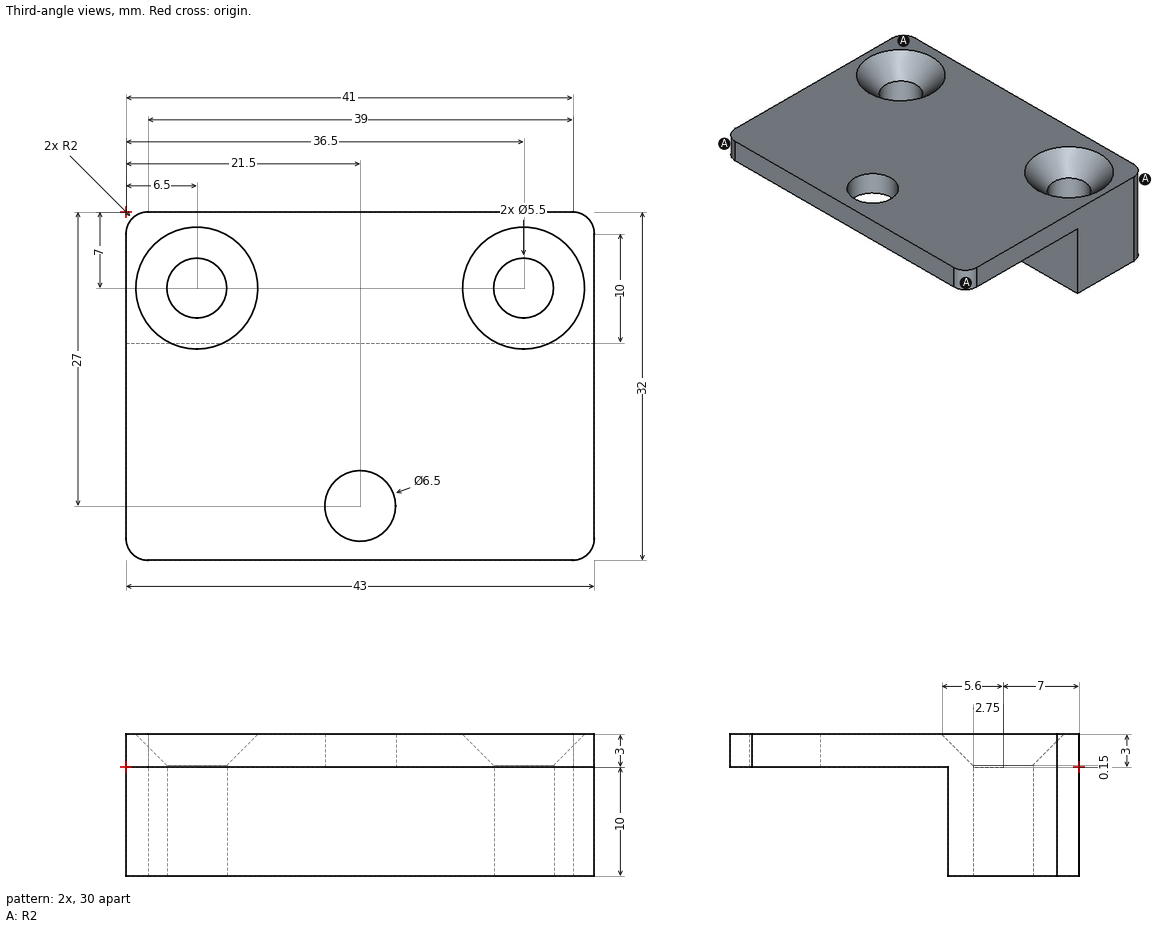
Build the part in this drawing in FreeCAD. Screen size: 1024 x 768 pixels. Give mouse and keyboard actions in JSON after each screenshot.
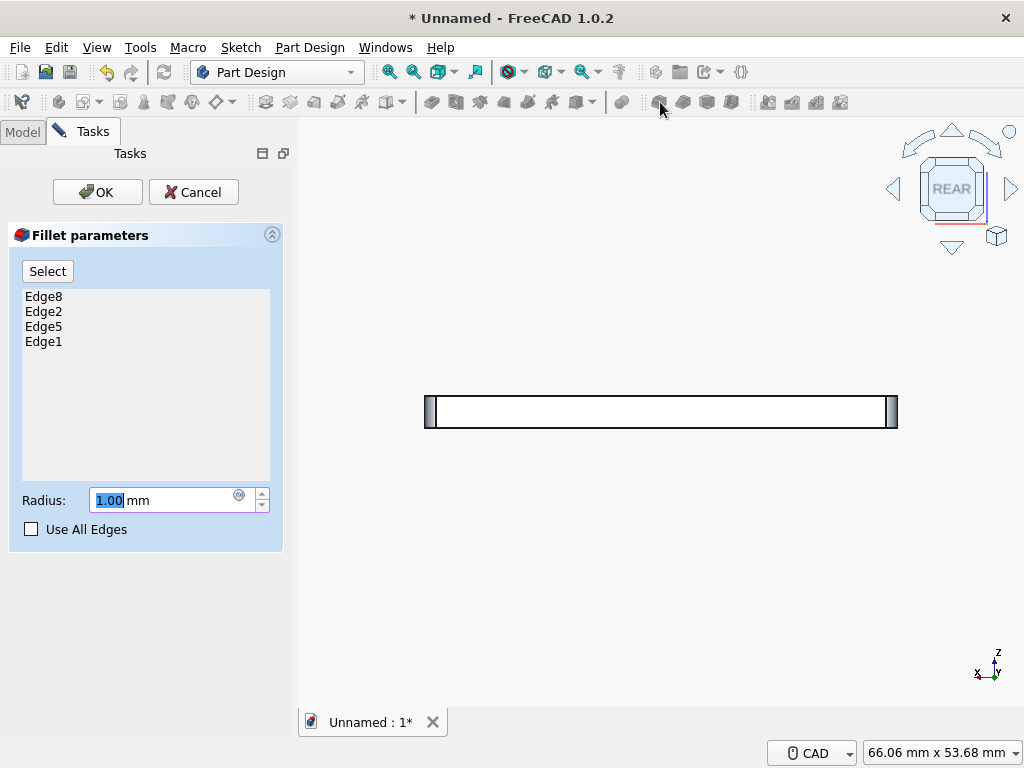
{"action": "type", "text": "2"}
{"action": "key", "text": "Tab"}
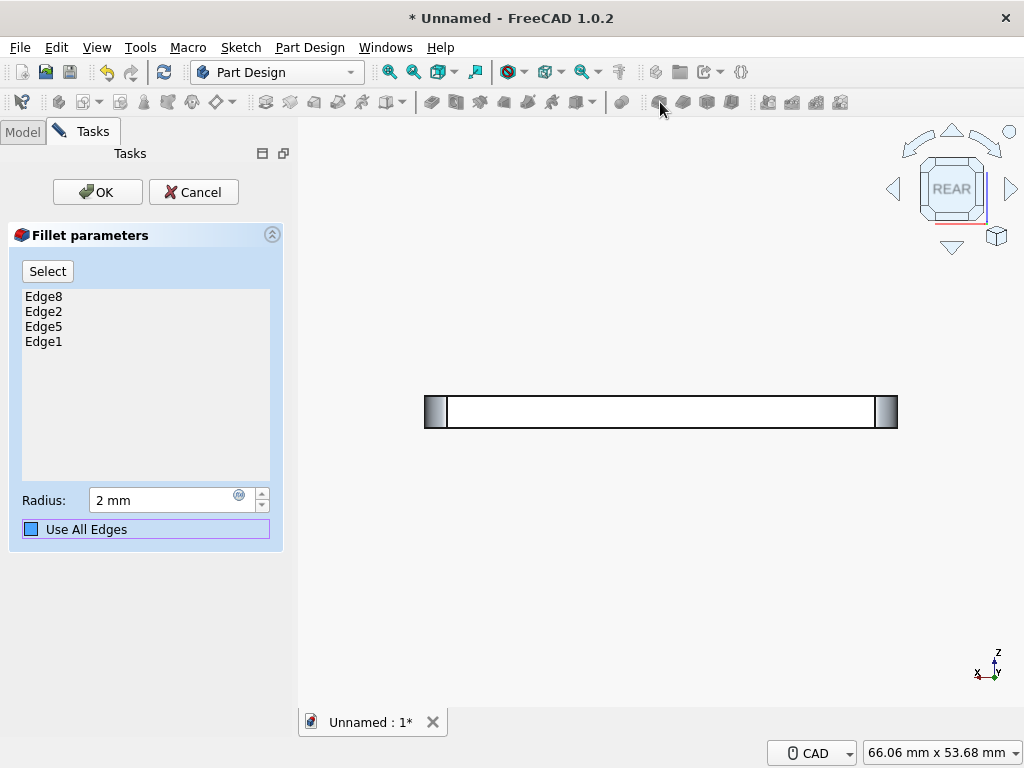
{"action": "left_click", "coordinate": [98, 192]}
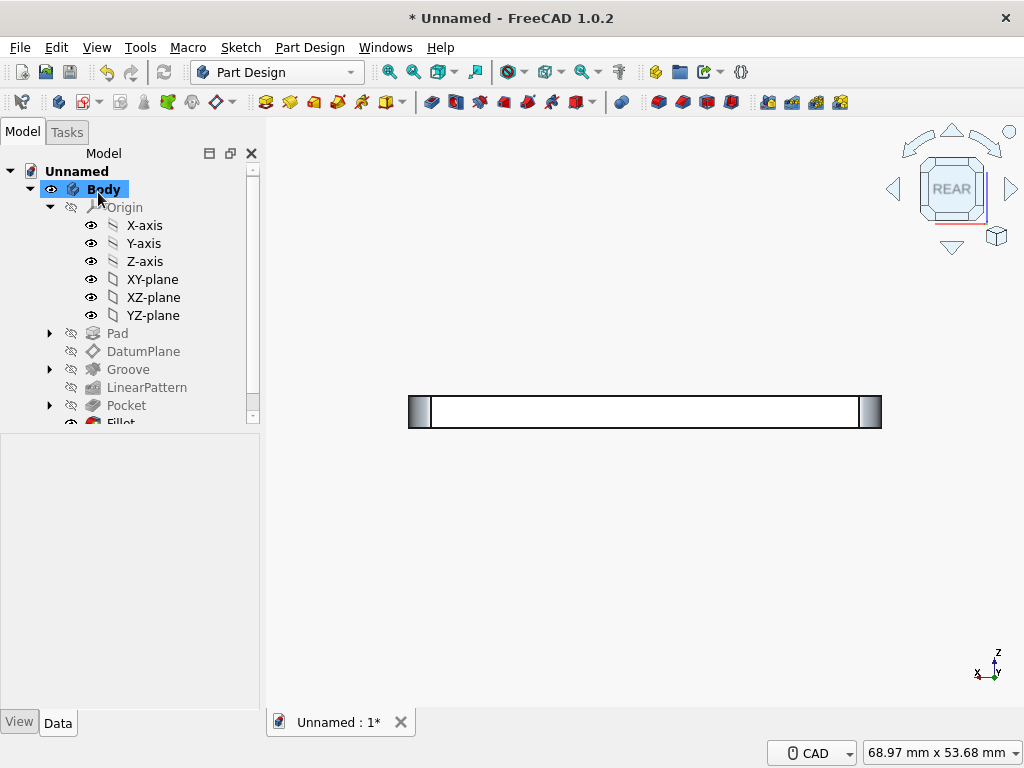
{"action": "left_click", "coordinate": [84, 102]}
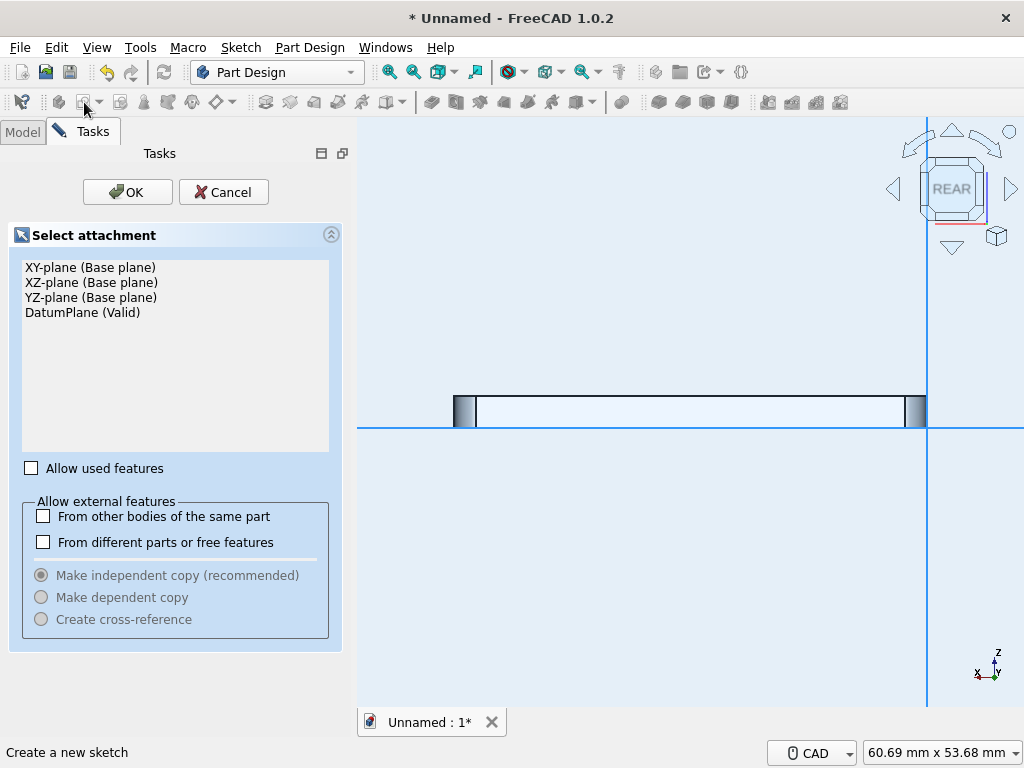
{"action": "left_click", "coordinate": [82, 268]}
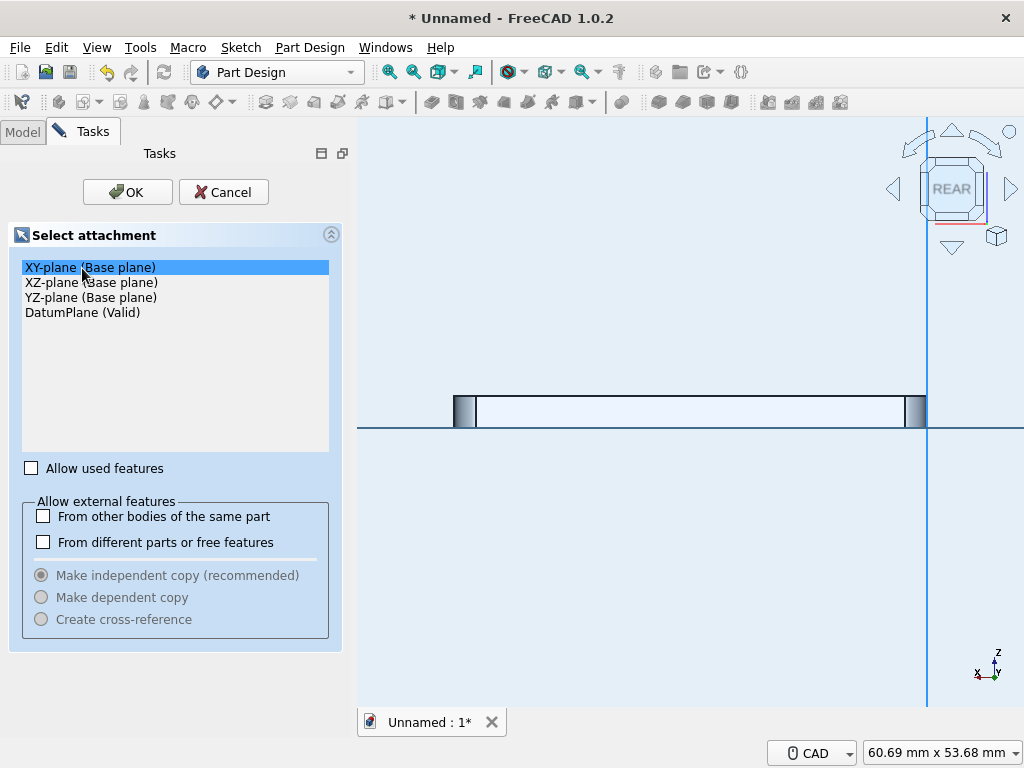
{"action": "left_click", "coordinate": [128, 192]}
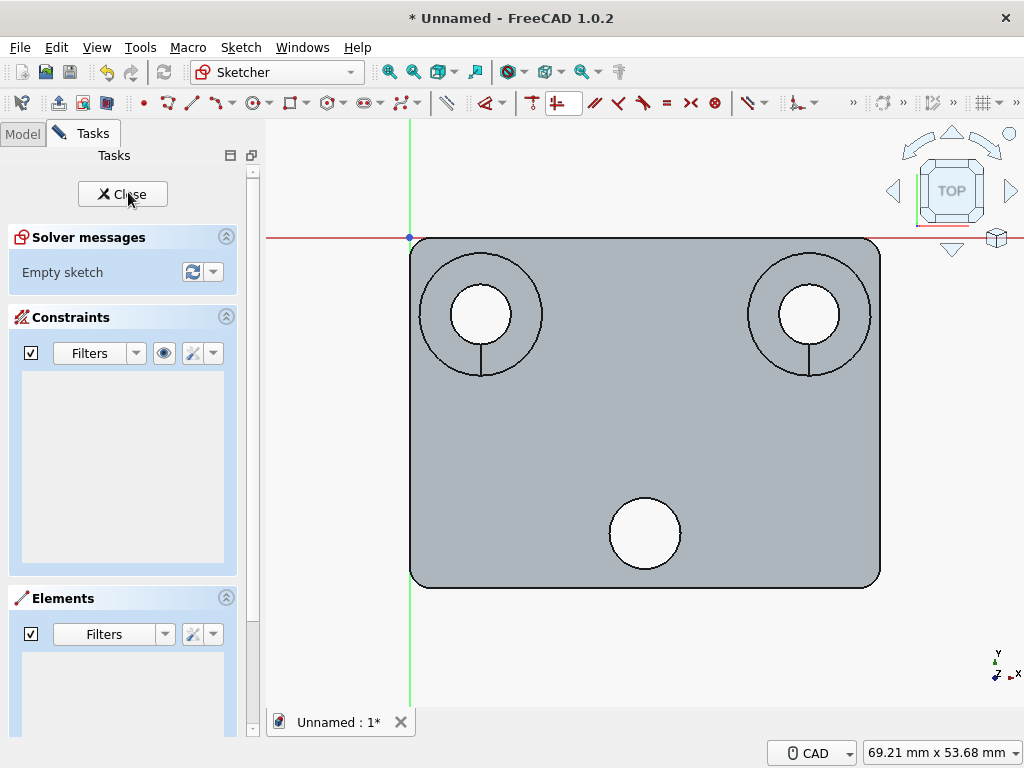
{"action": "left_click", "coordinate": [108, 104]}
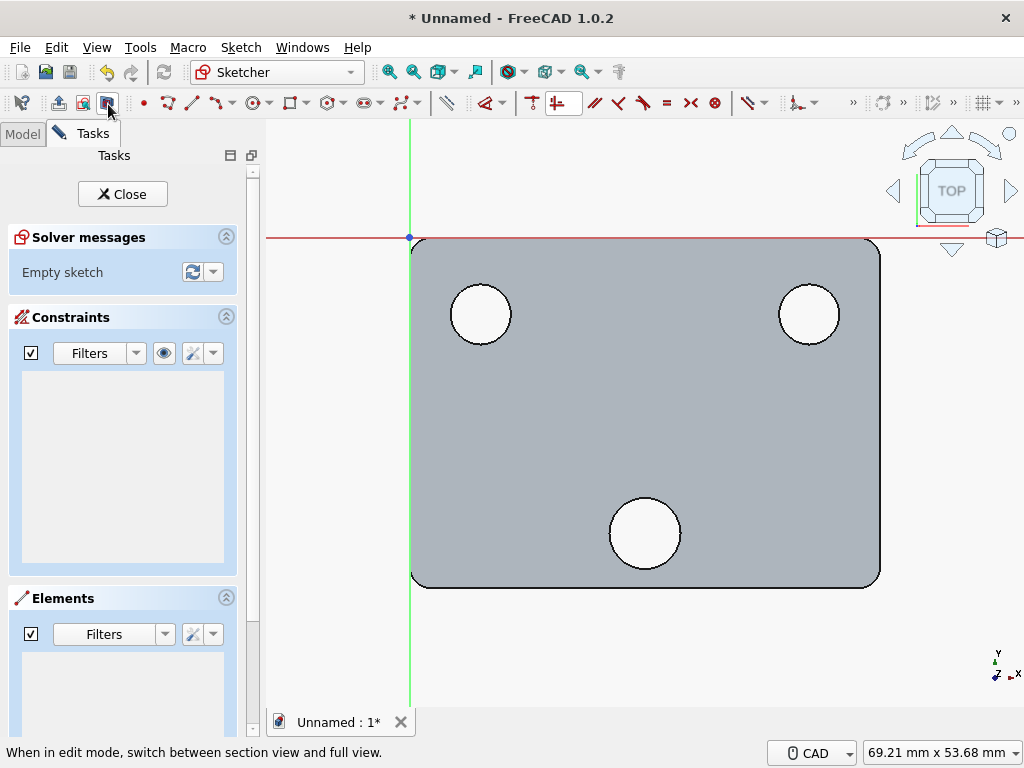
{"action": "scroll", "coordinate": [294, 679], "scroll_direction": "down", "scroll_amount": 1}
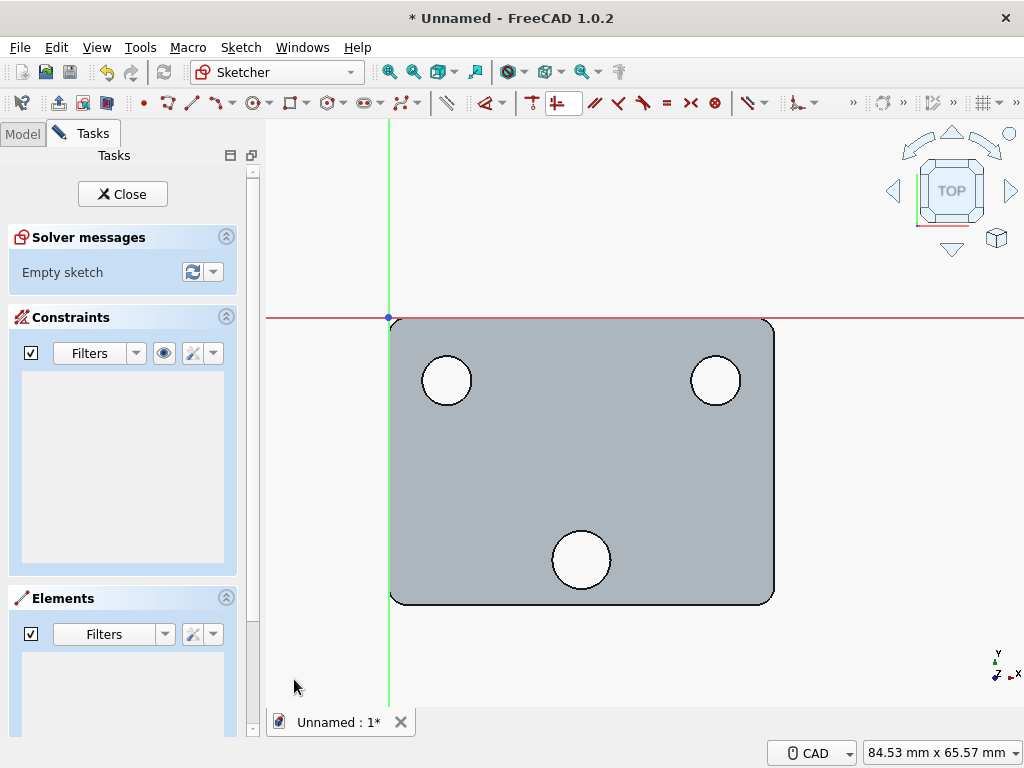
{"action": "key", "text": "g m"}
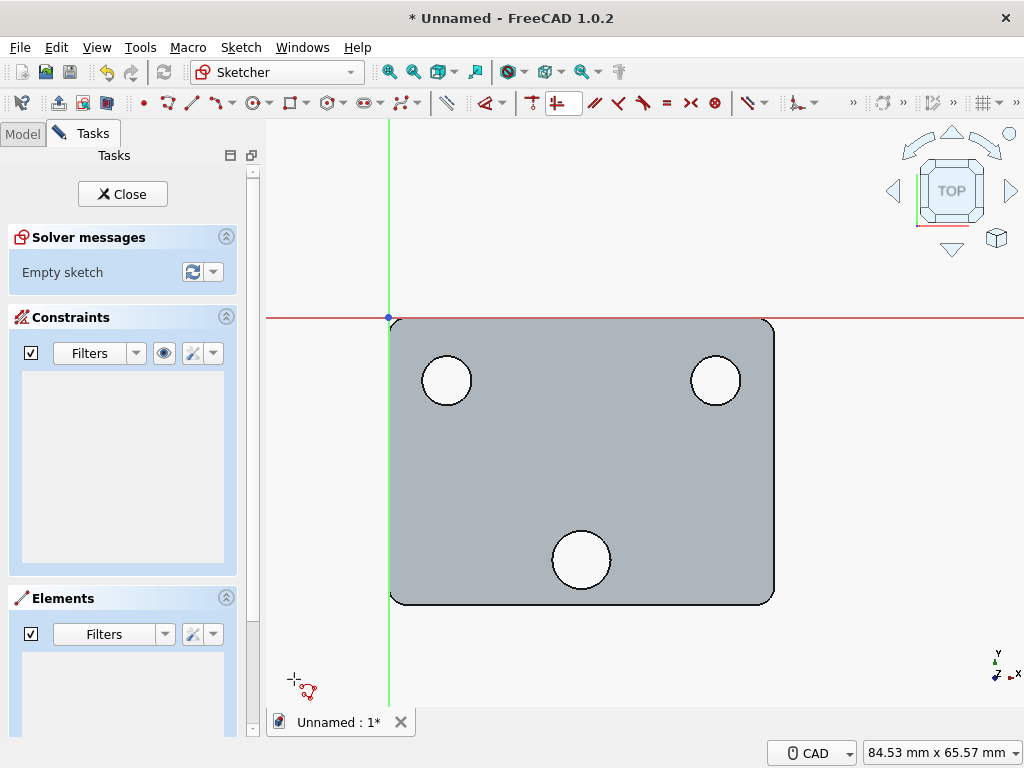
{"action": "left_click", "coordinate": [774, 336]}
{"action": "left_click", "coordinate": [774, 426]}
{"action": "left_click", "coordinate": [389, 426]}
{"action": "left_click", "coordinate": [398, 336]}
{"action": "right_click", "coordinate": [398, 336]}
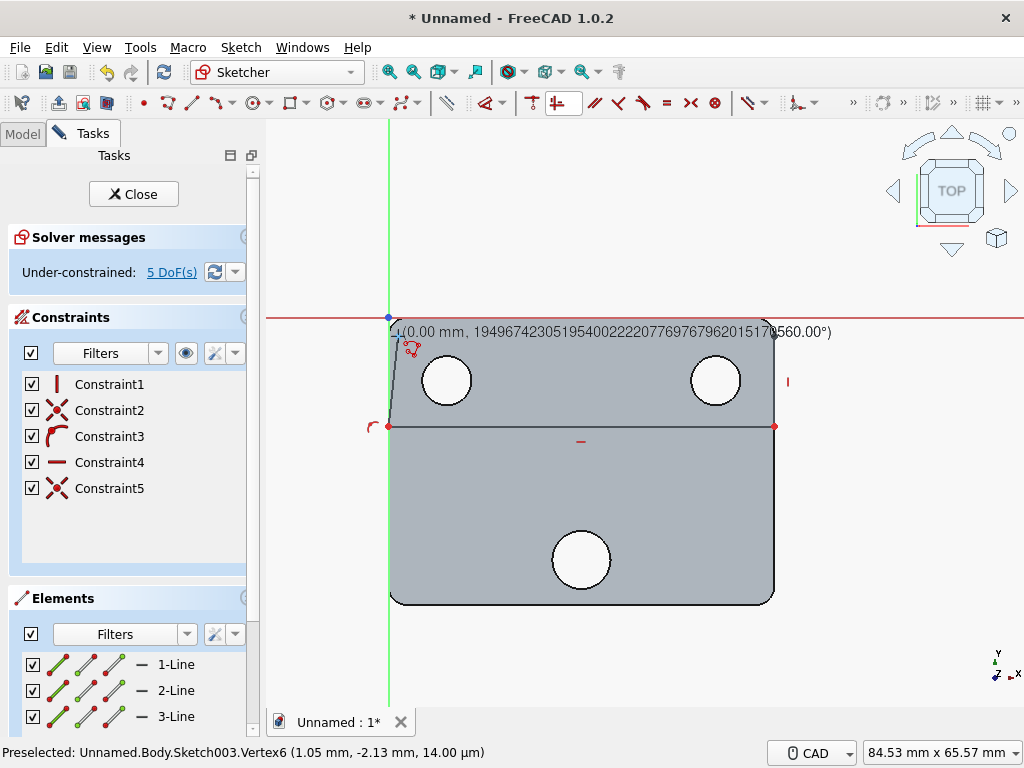
{"action": "left_click", "coordinate": [192, 104]}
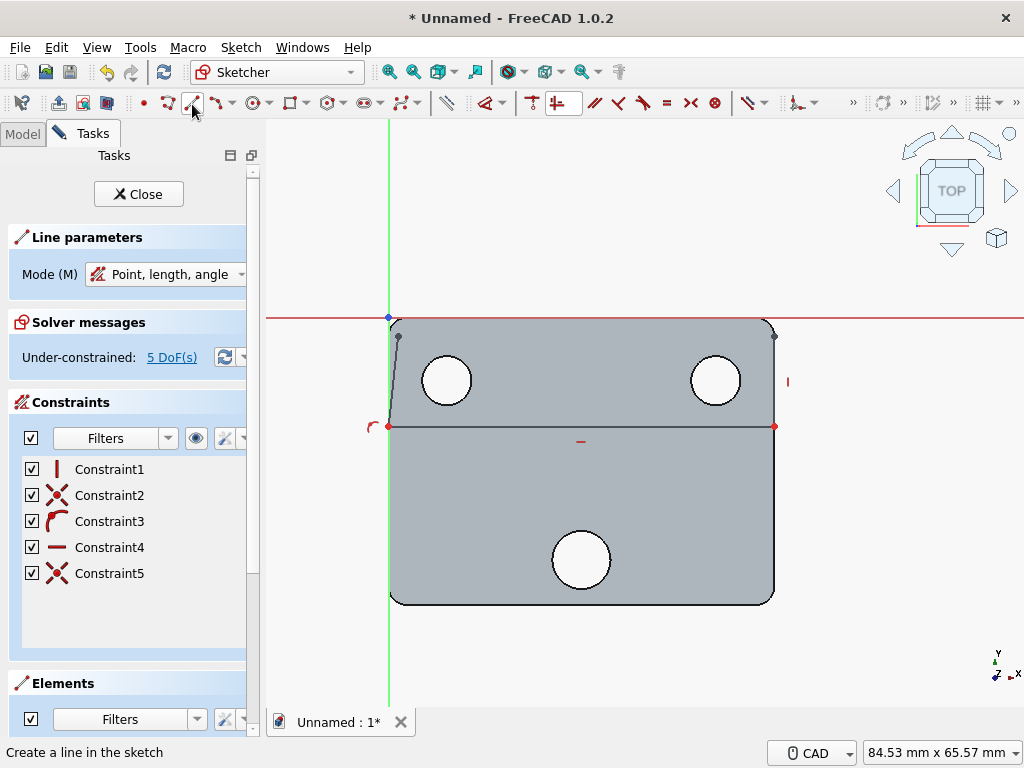
{"action": "left_click", "coordinate": [407, 318]}
{"action": "left_click", "coordinate": [756, 327]}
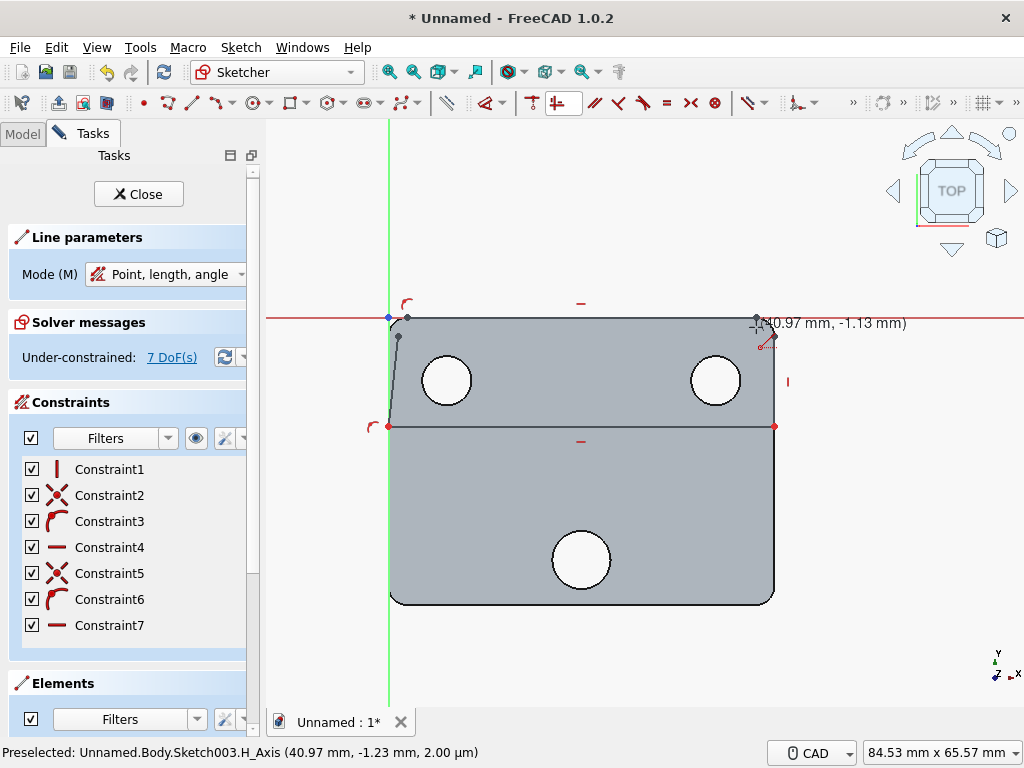
{"action": "left_click", "coordinate": [216, 104]}